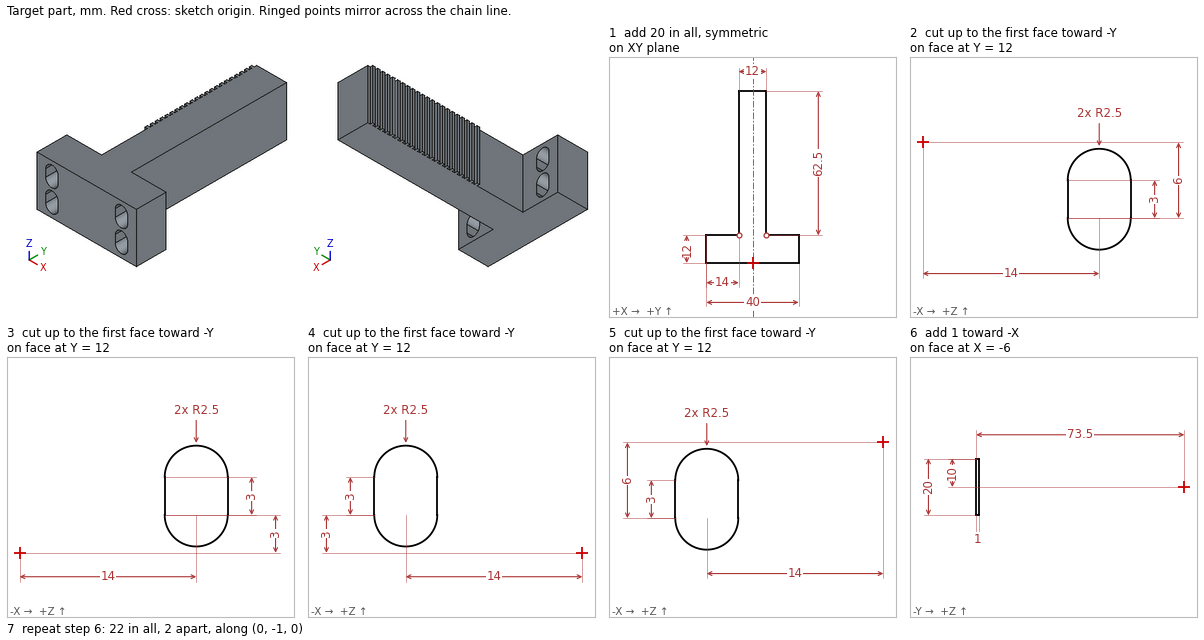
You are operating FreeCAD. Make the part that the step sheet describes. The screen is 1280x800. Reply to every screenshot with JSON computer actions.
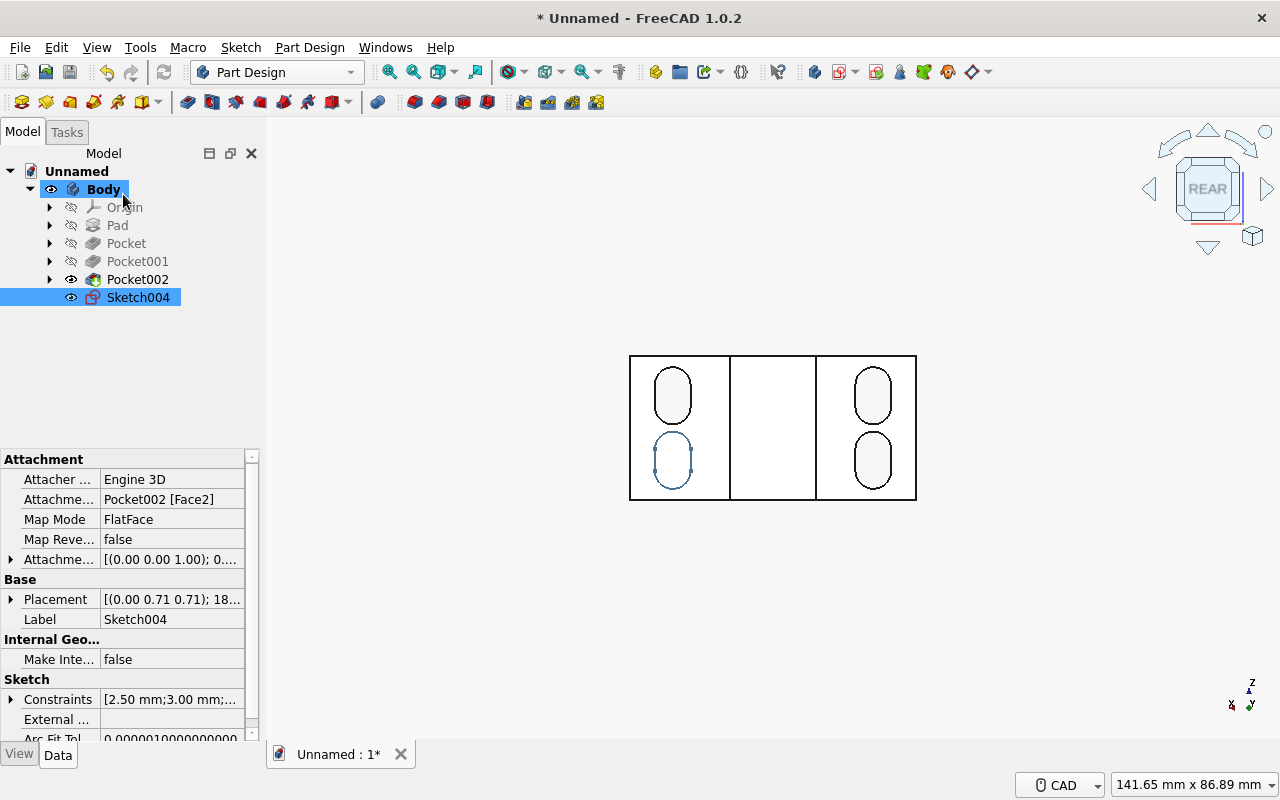
{"action": "left_click", "coordinate": [188, 102]}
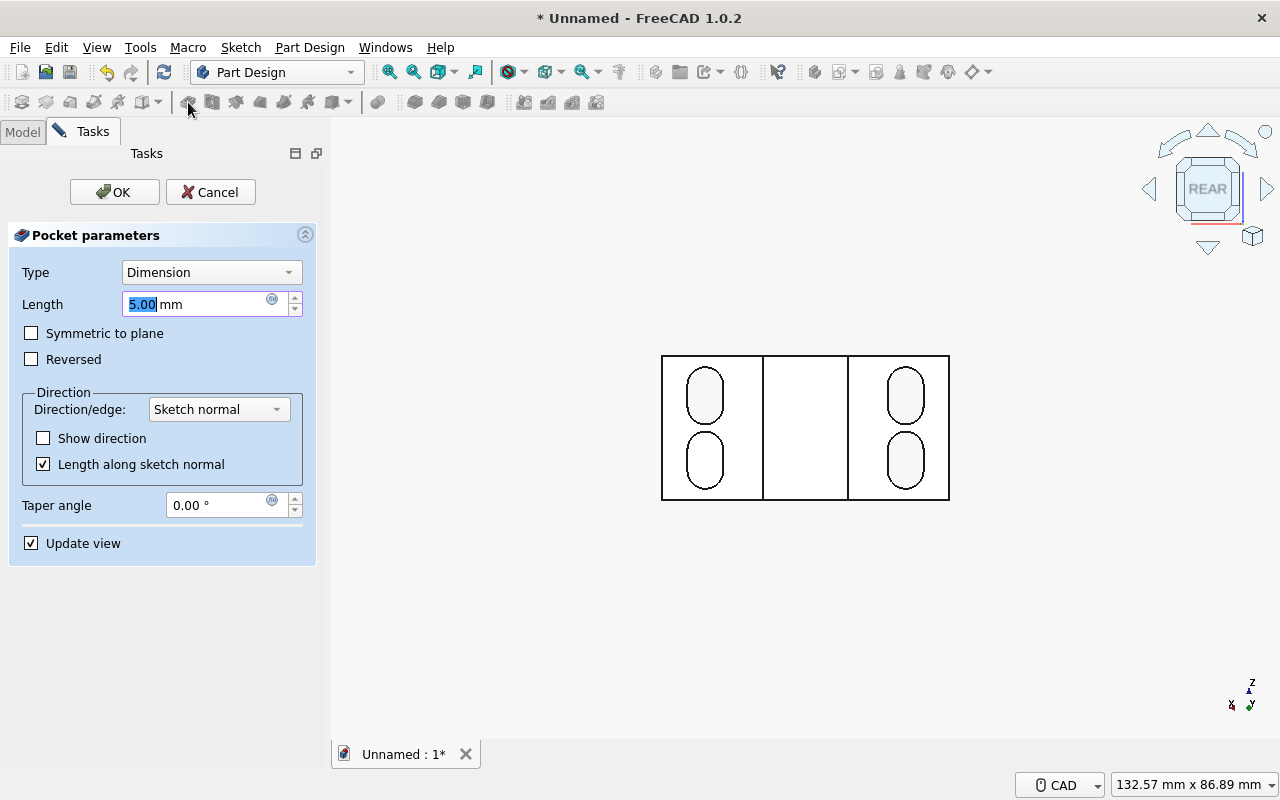
{"action": "left_click", "coordinate": [212, 272]}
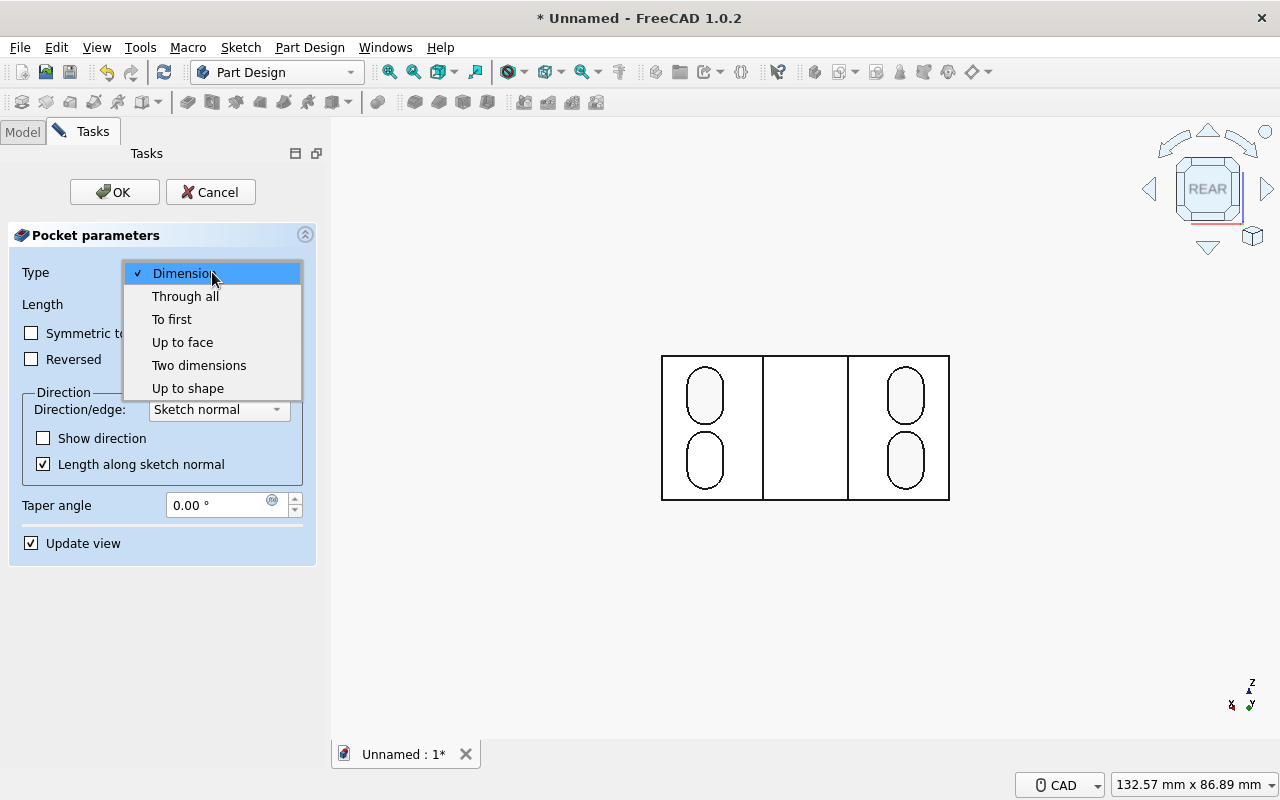
{"action": "left_click", "coordinate": [212, 320]}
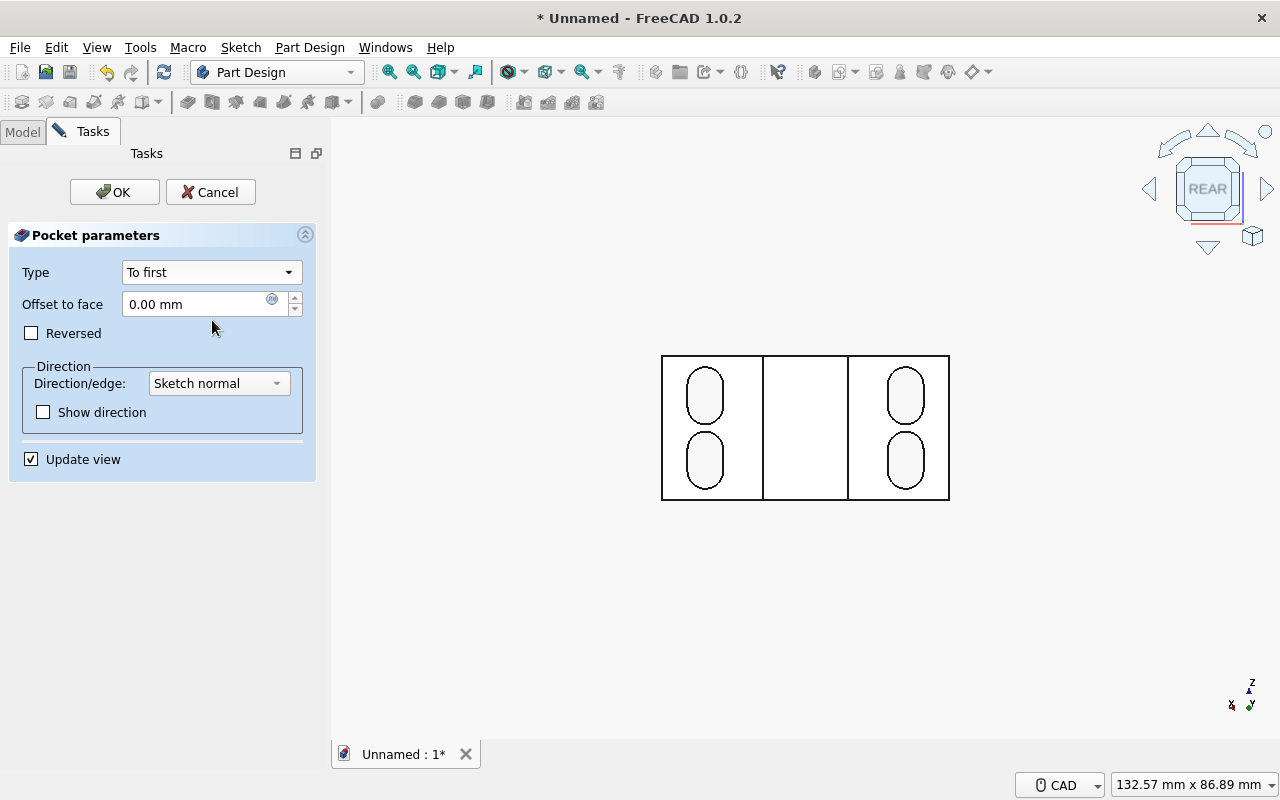
{"action": "left_click", "coordinate": [115, 192]}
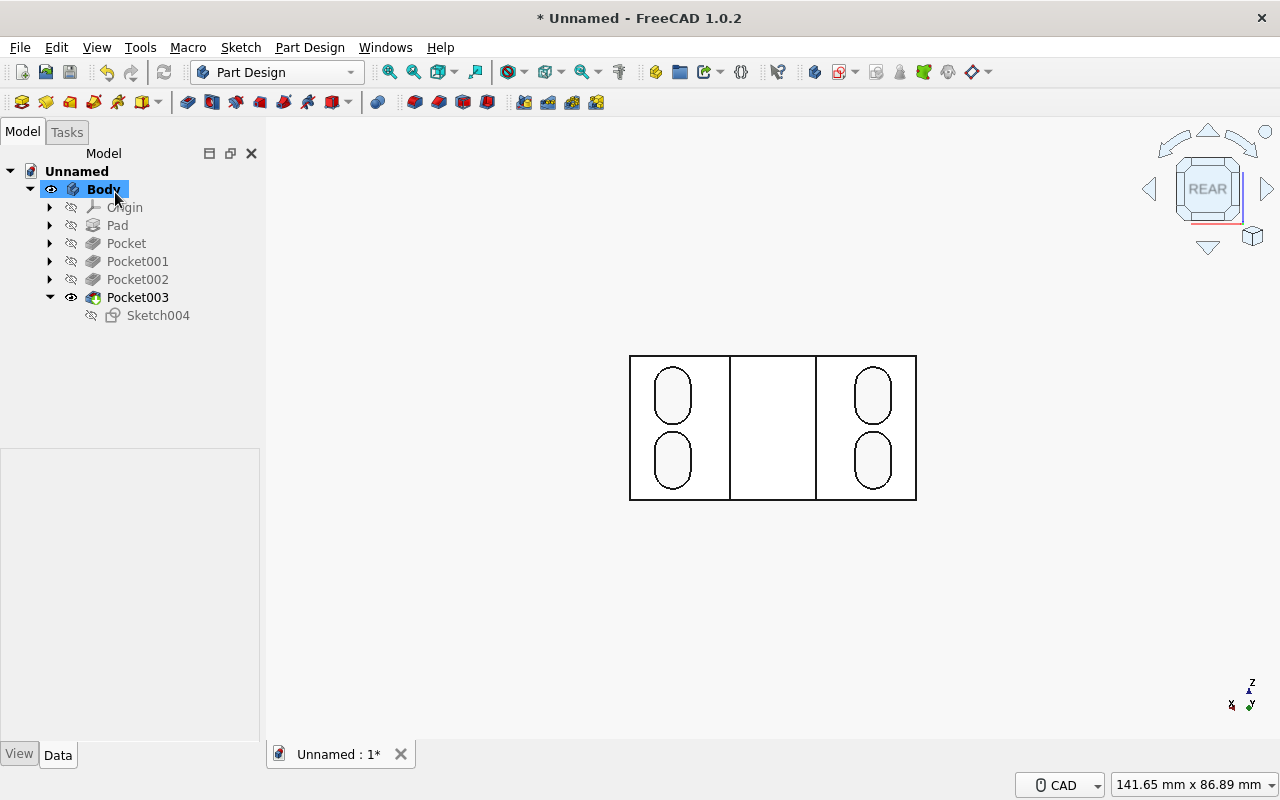
{"action": "key", "text": "v f"}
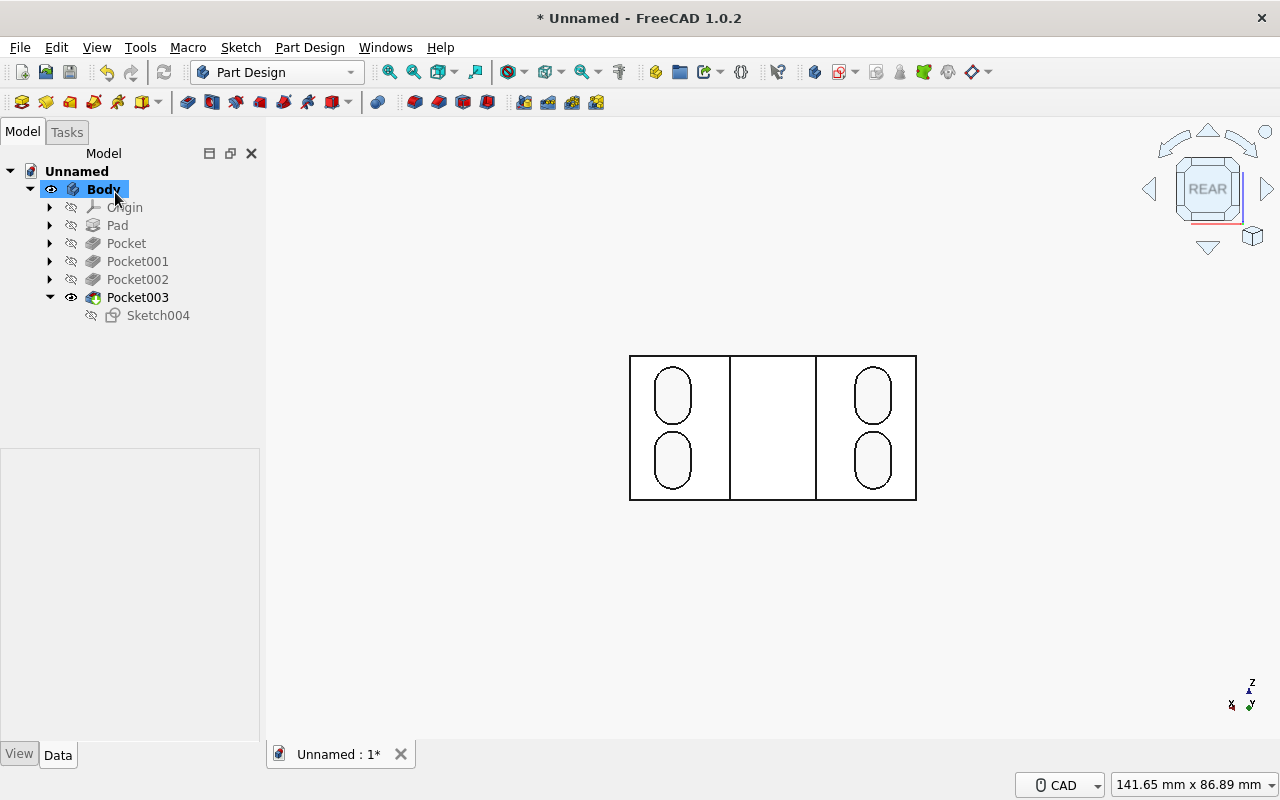
{"action": "key", "text": "6"}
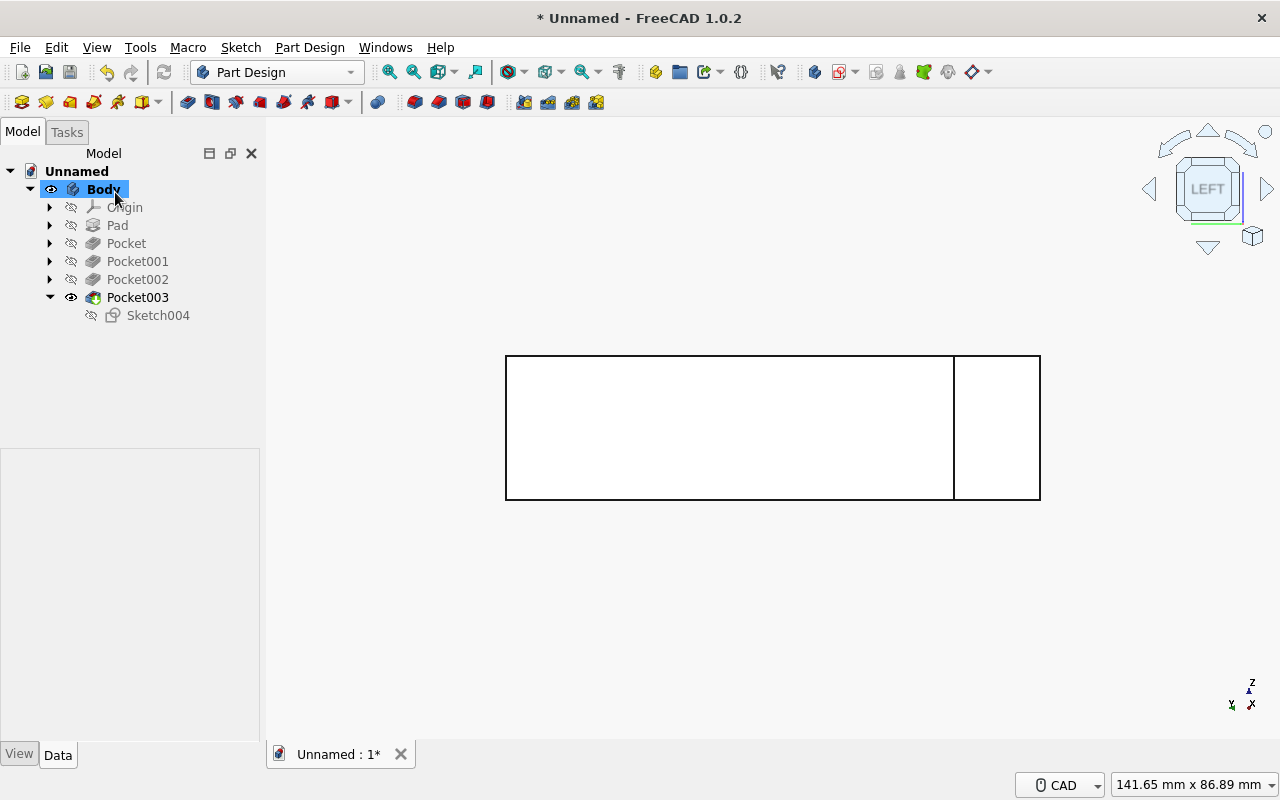
{"action": "left_click", "coordinate": [602, 427]}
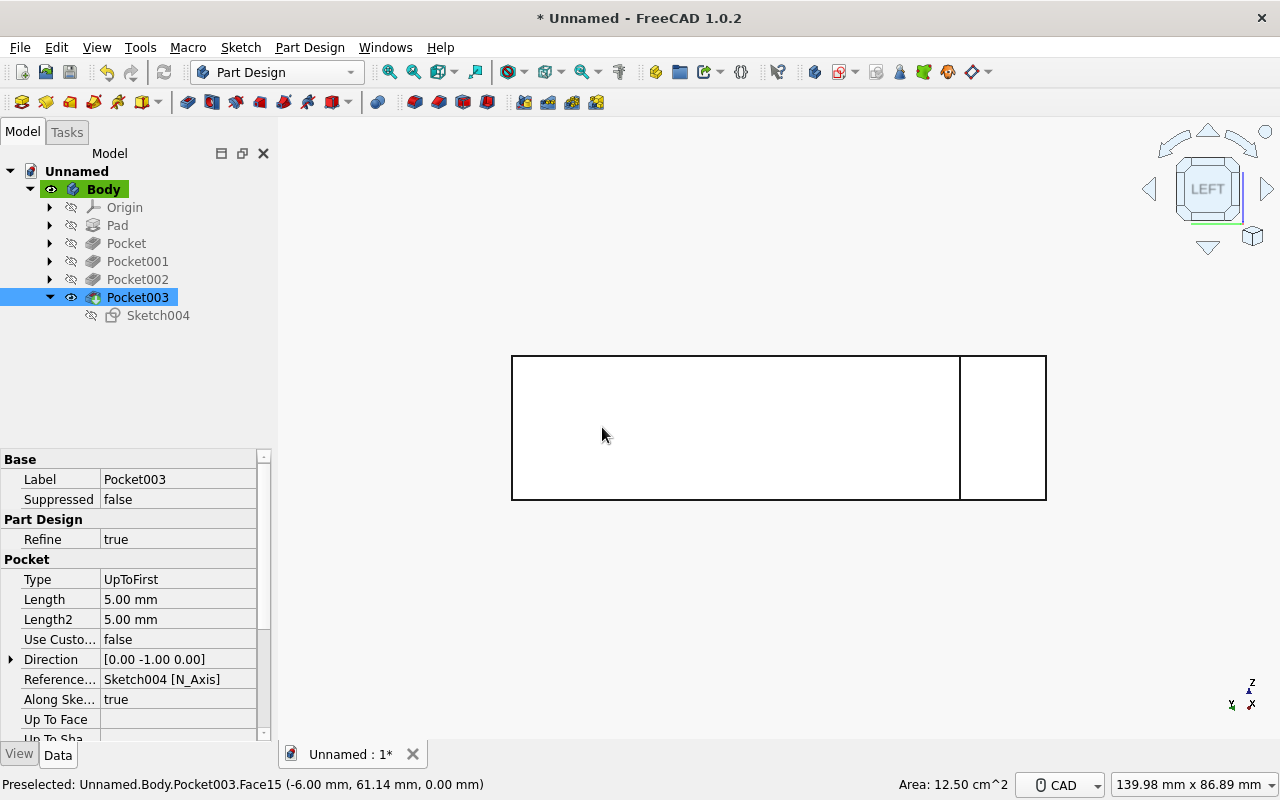
{"action": "left_click", "coordinate": [840, 72]}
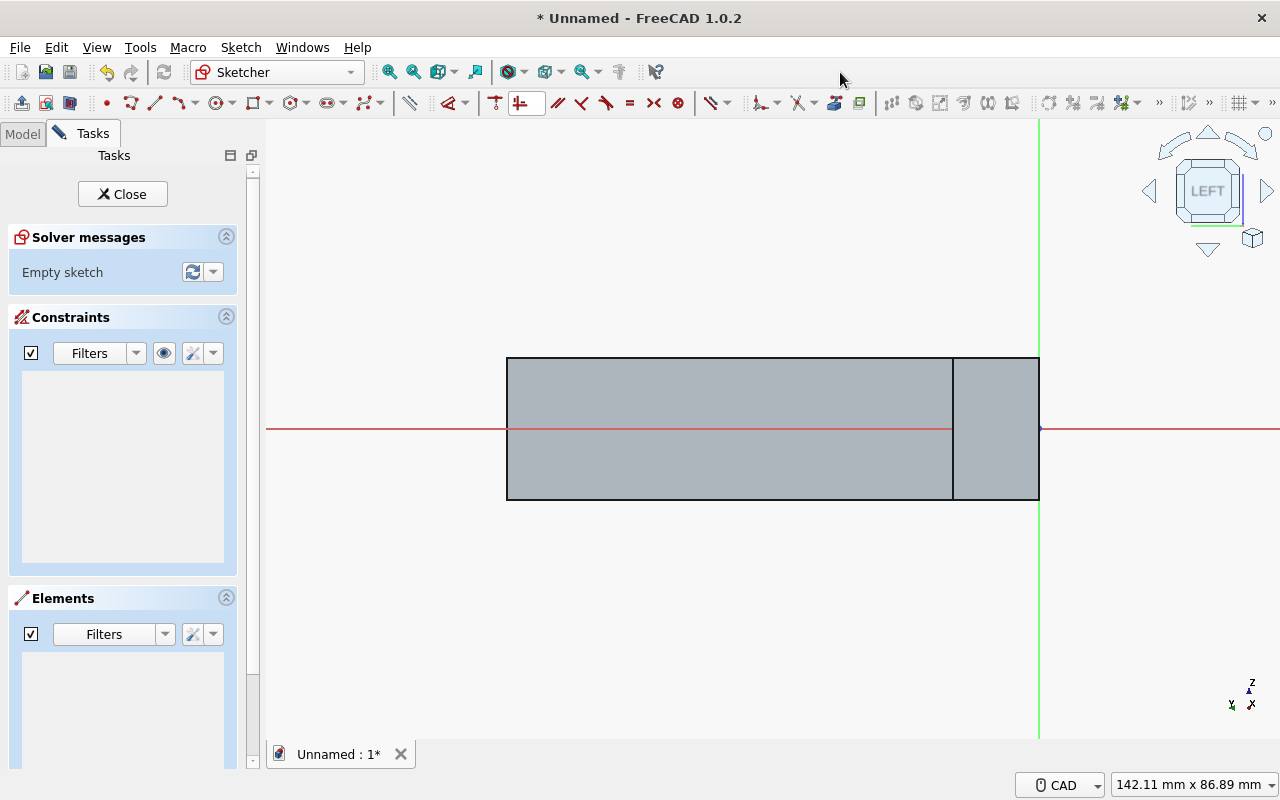
{"action": "key", "text": "q s"}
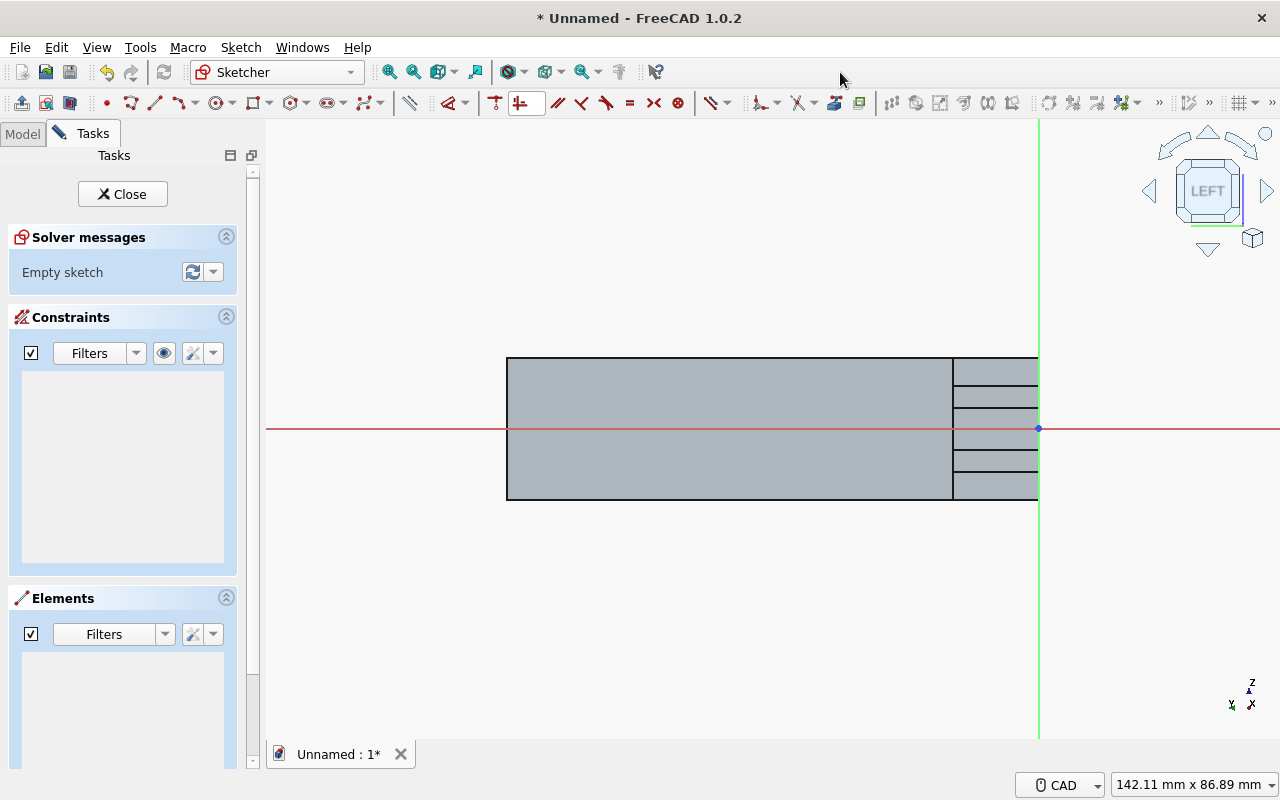
{"action": "scroll", "coordinate": [409, 429], "scroll_direction": "up", "scroll_amount": 5}